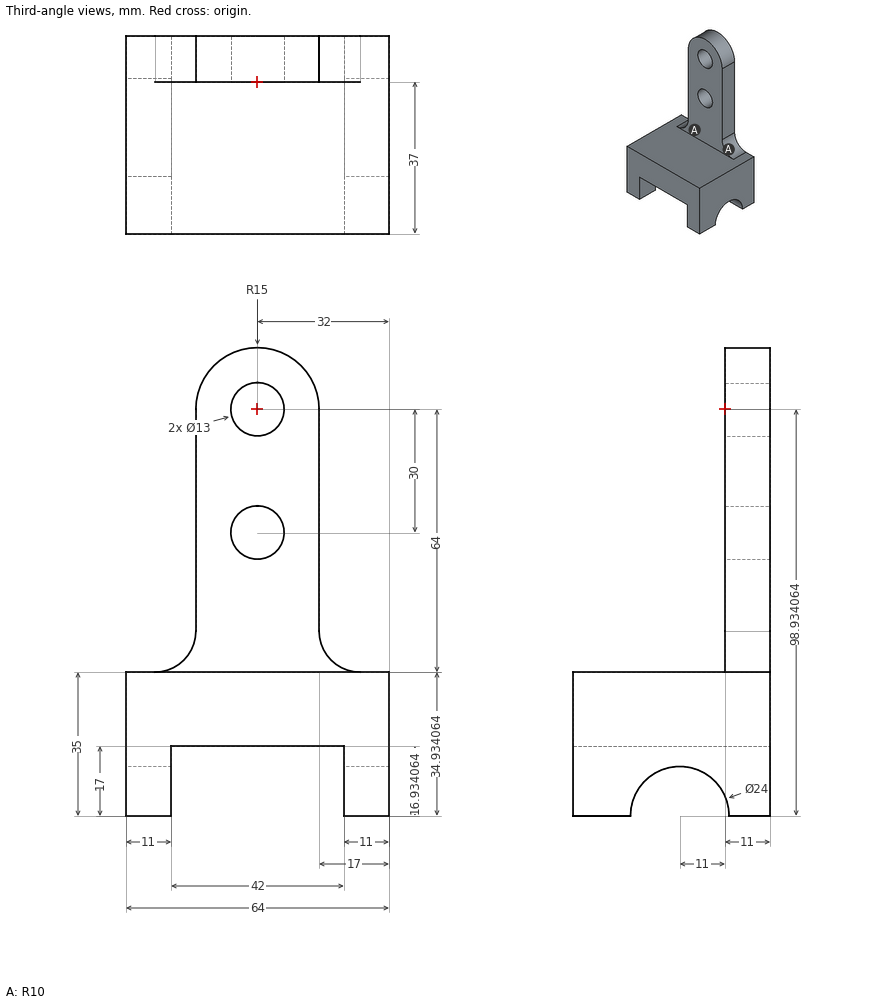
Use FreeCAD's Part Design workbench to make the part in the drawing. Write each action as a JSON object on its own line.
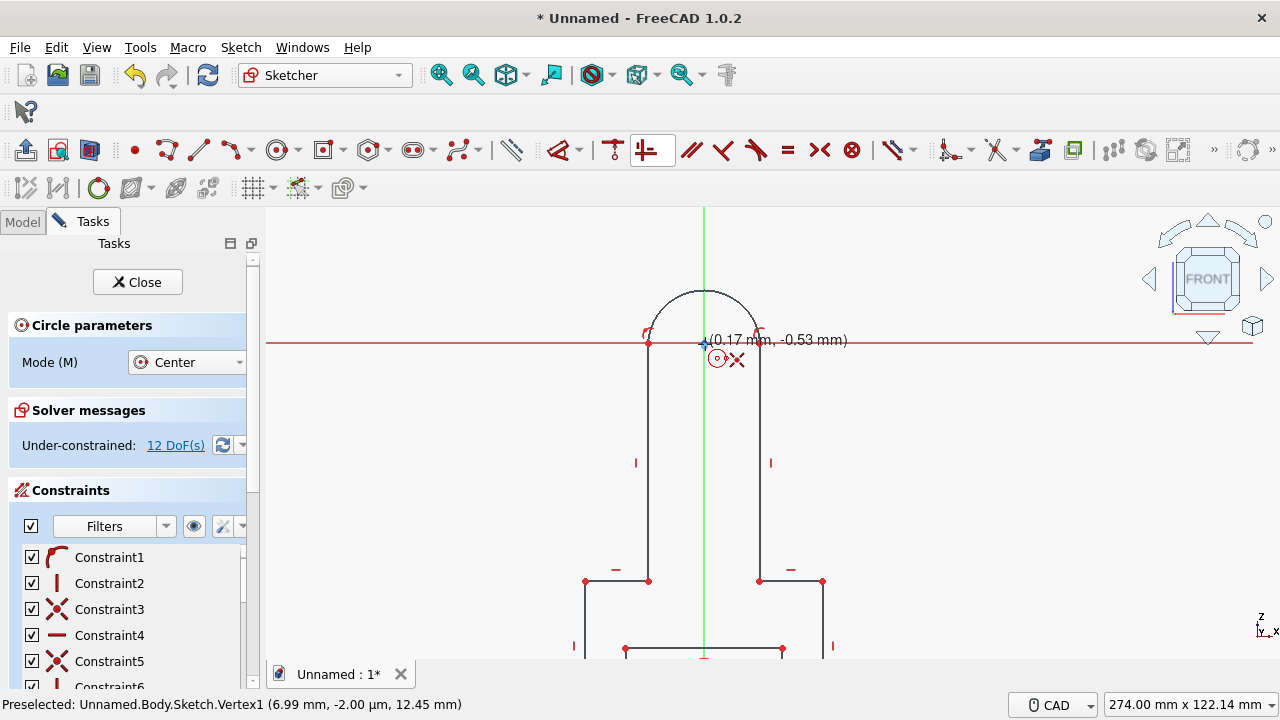
{"action": "left_click", "coordinate": [704, 343]}
{"action": "left_click", "coordinate": [721, 326]}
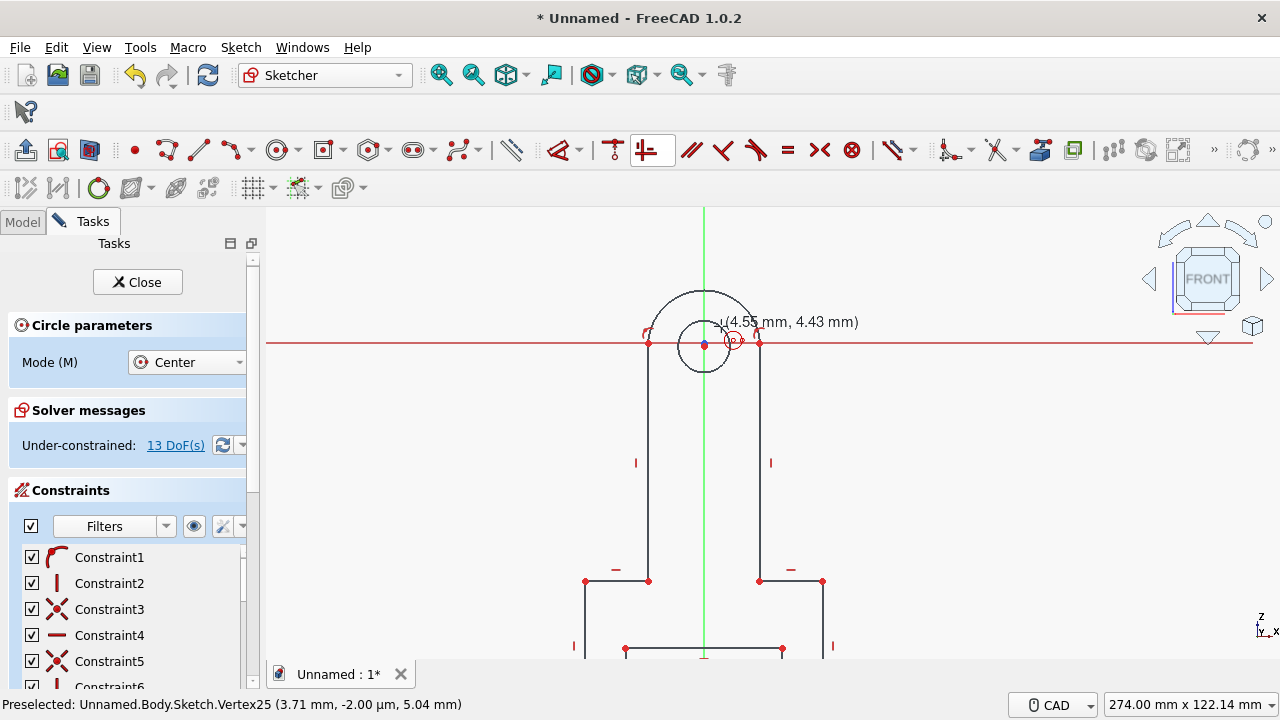
{"action": "left_click", "coordinate": [704, 454]}
{"action": "left_click", "coordinate": [721, 437]}
{"action": "key", "text": "Escape"}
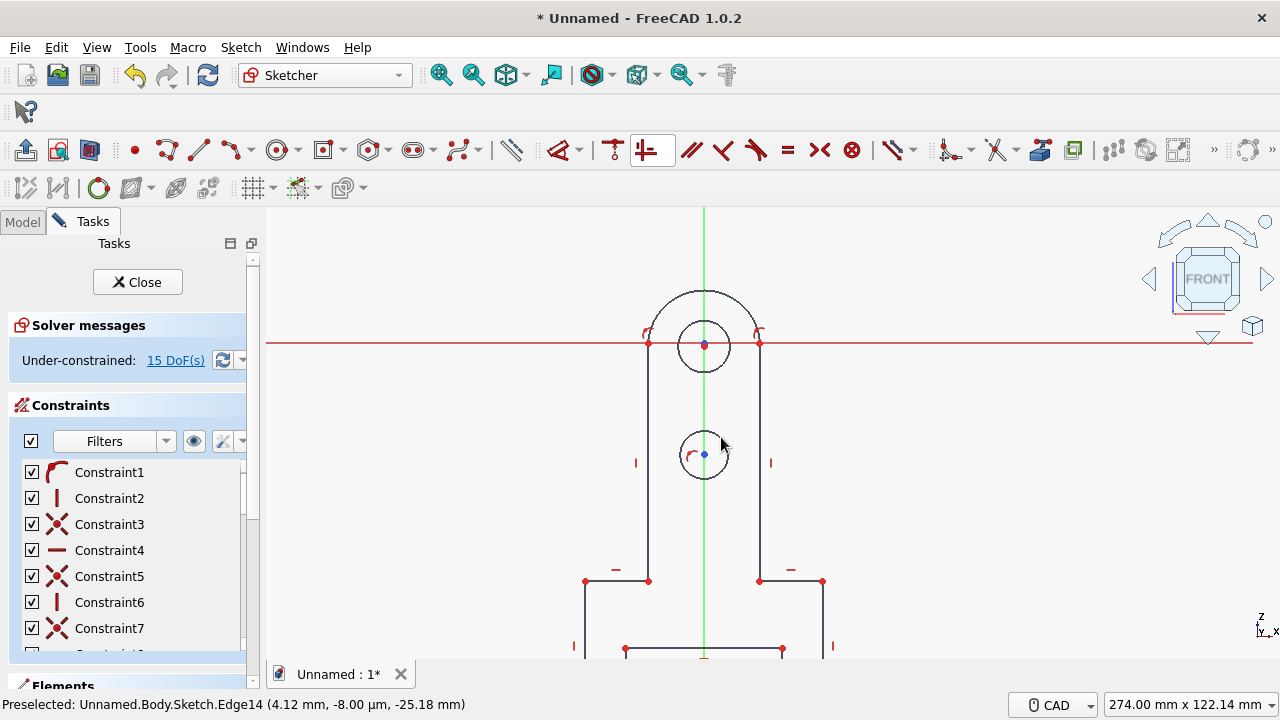
{"action": "left_click", "coordinate": [760, 415]}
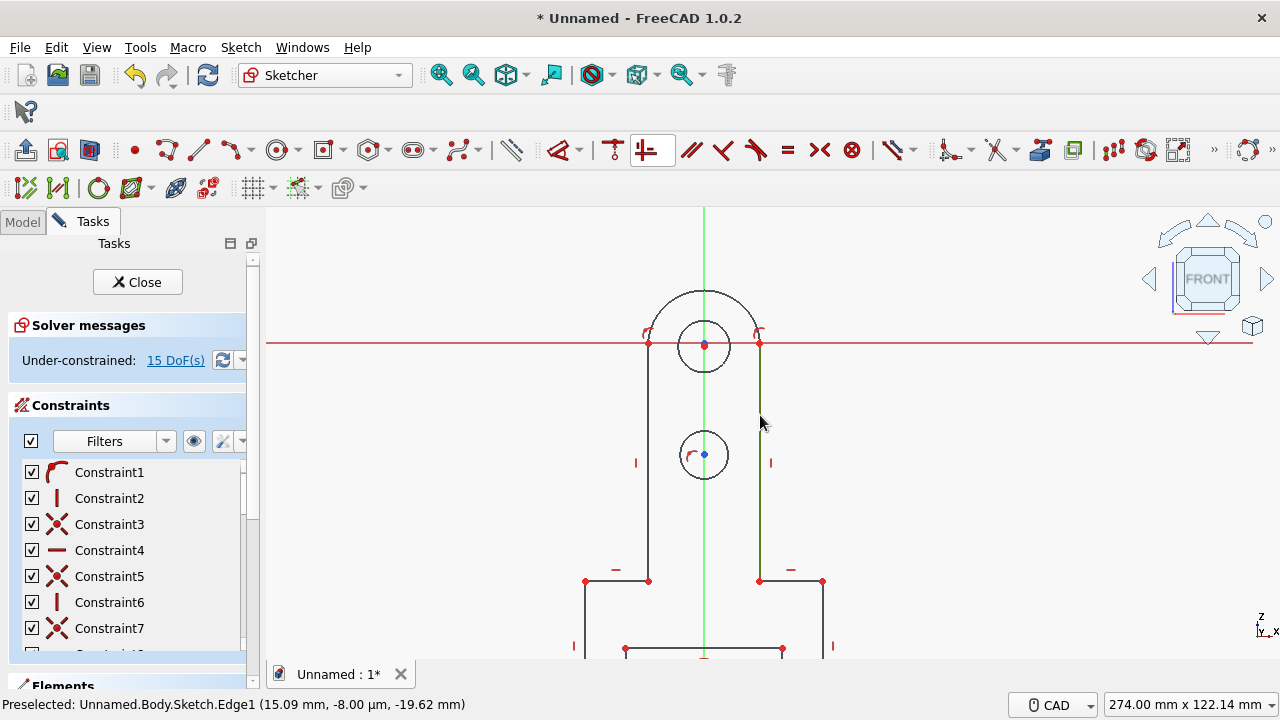
{"action": "left_click", "coordinate": [736, 300]}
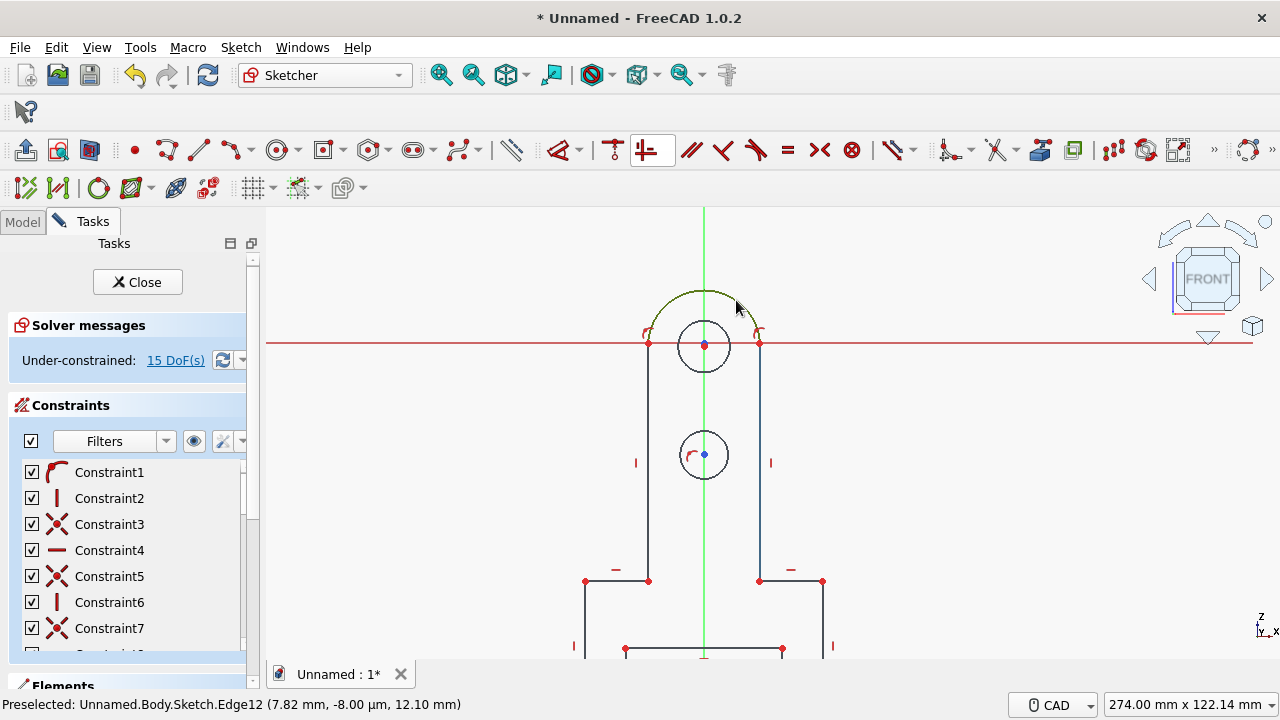
{"action": "left_click", "coordinate": [756, 150]}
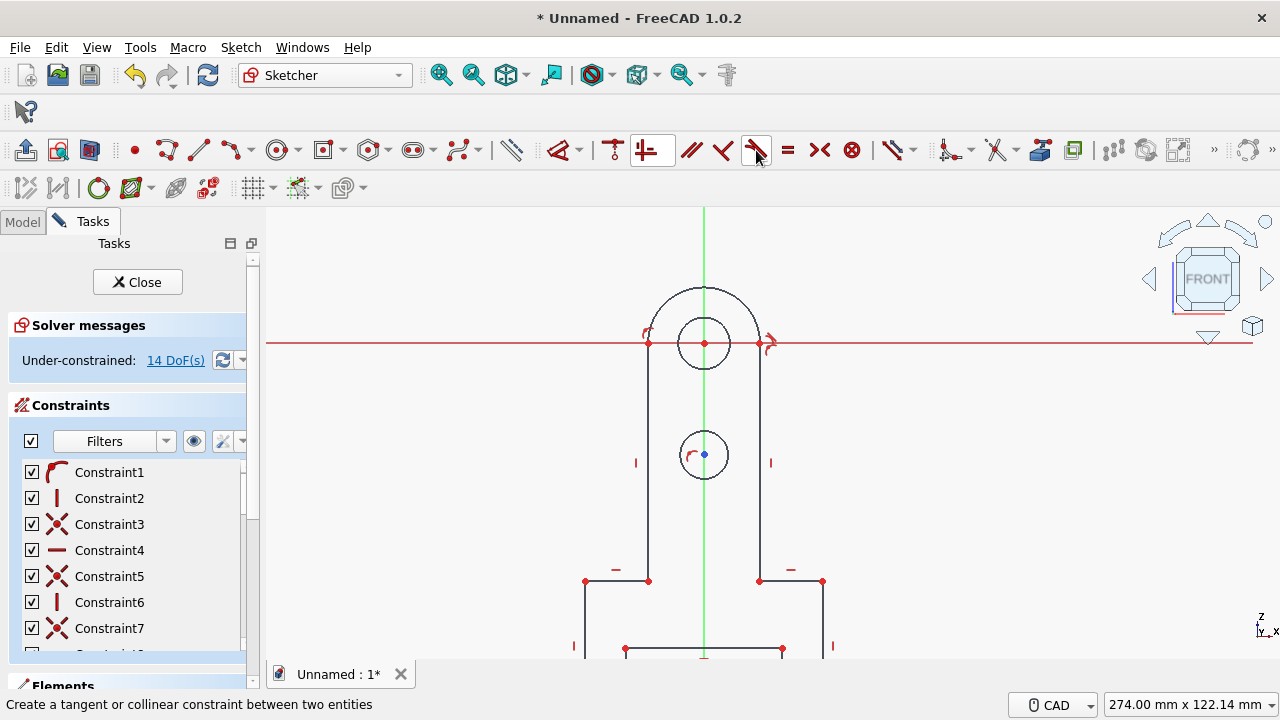
{"action": "left_click", "coordinate": [722, 325]}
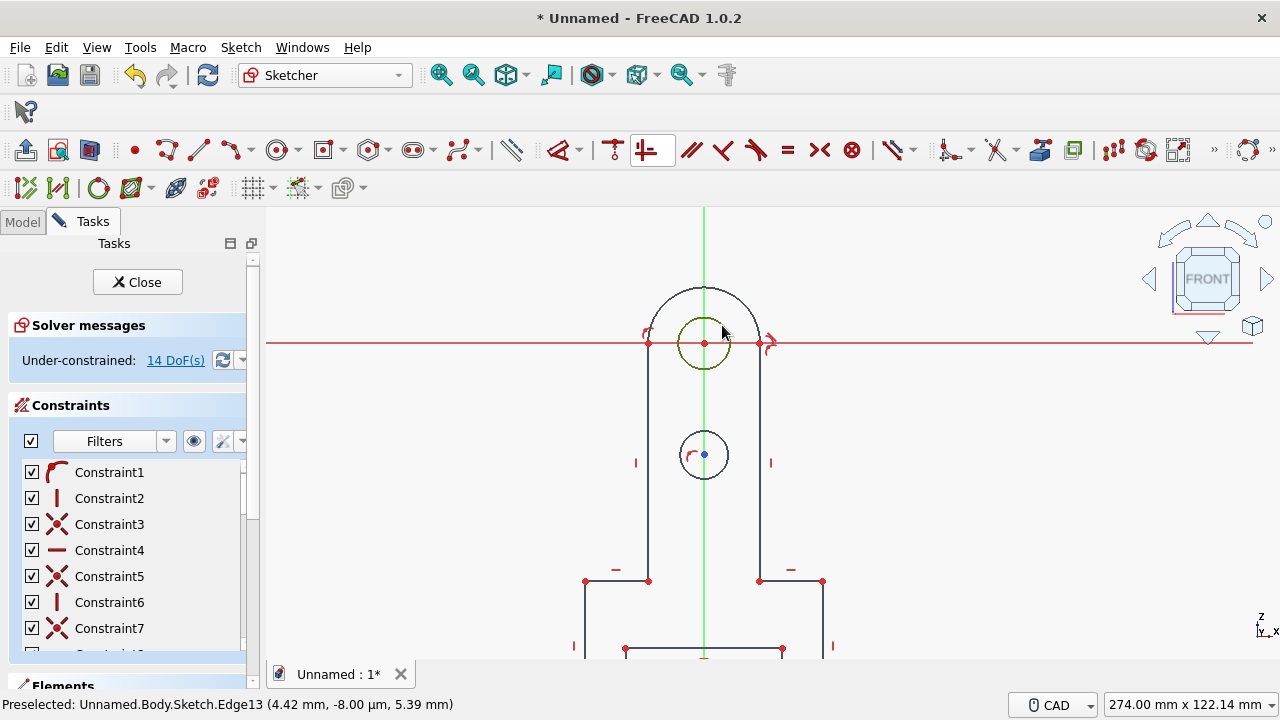
{"action": "left_click", "coordinate": [721, 438]}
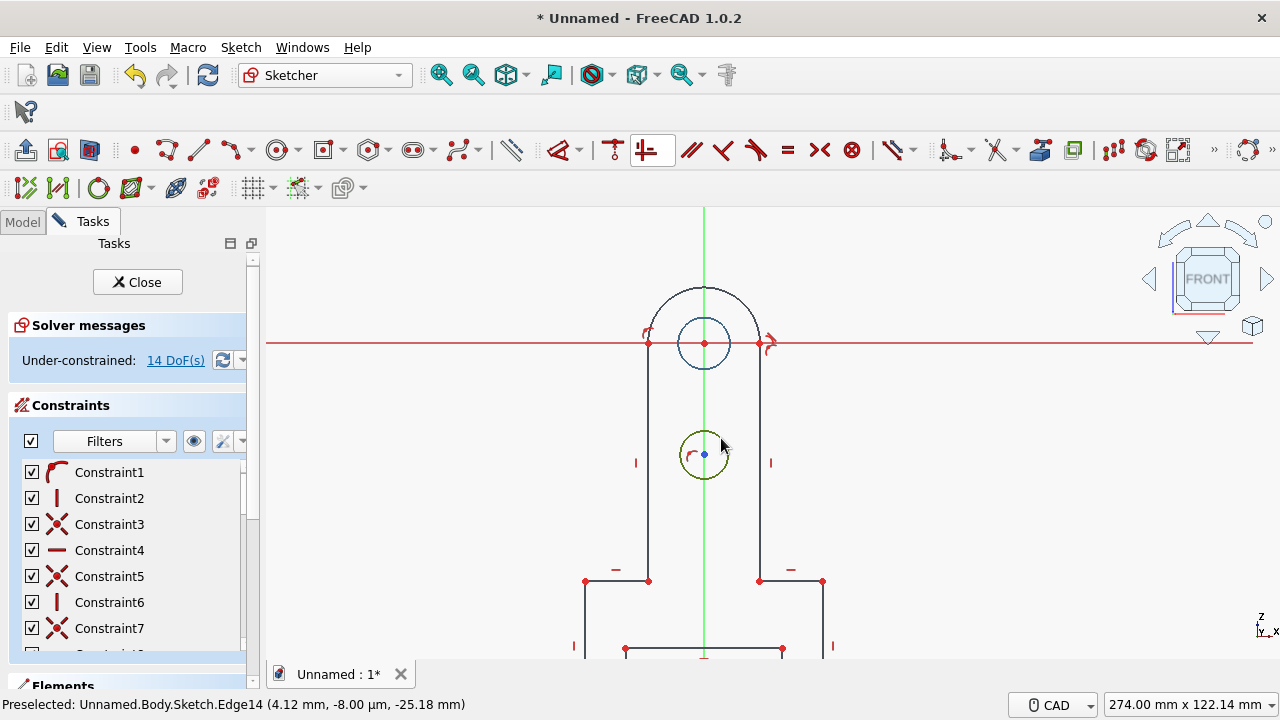
{"action": "left_click", "coordinate": [788, 150]}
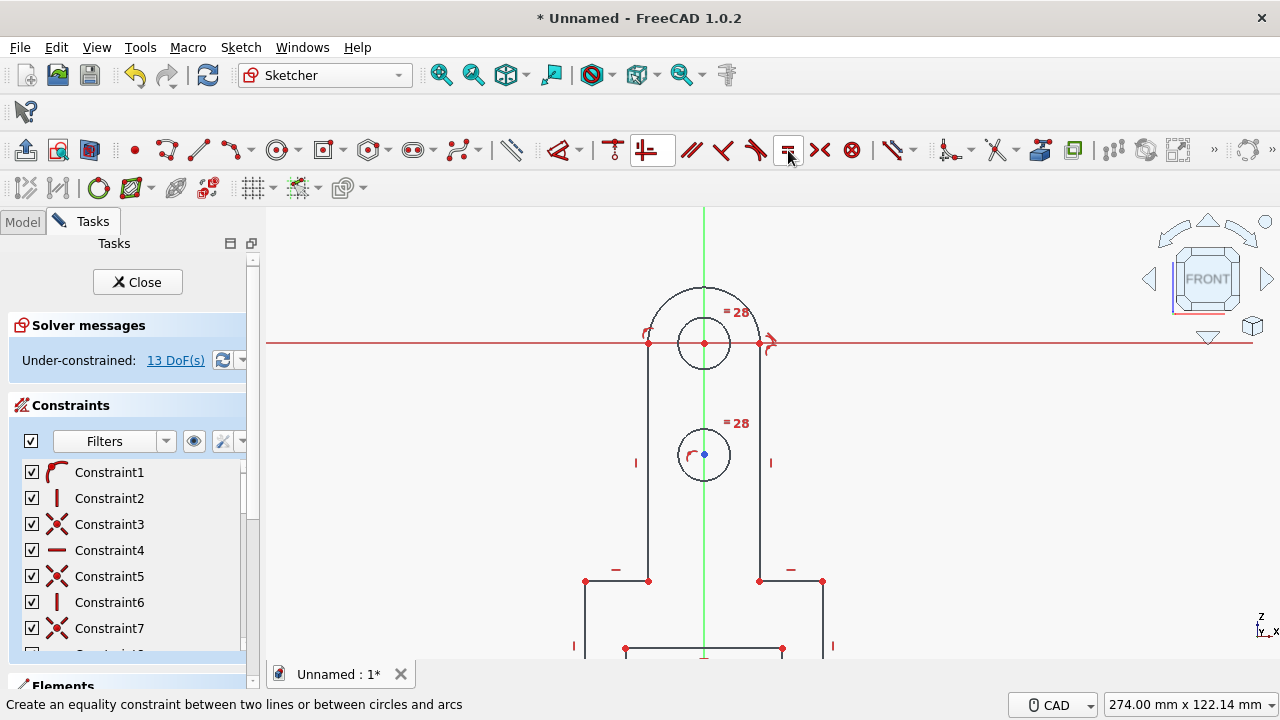
{"action": "left_click", "coordinate": [704, 343]}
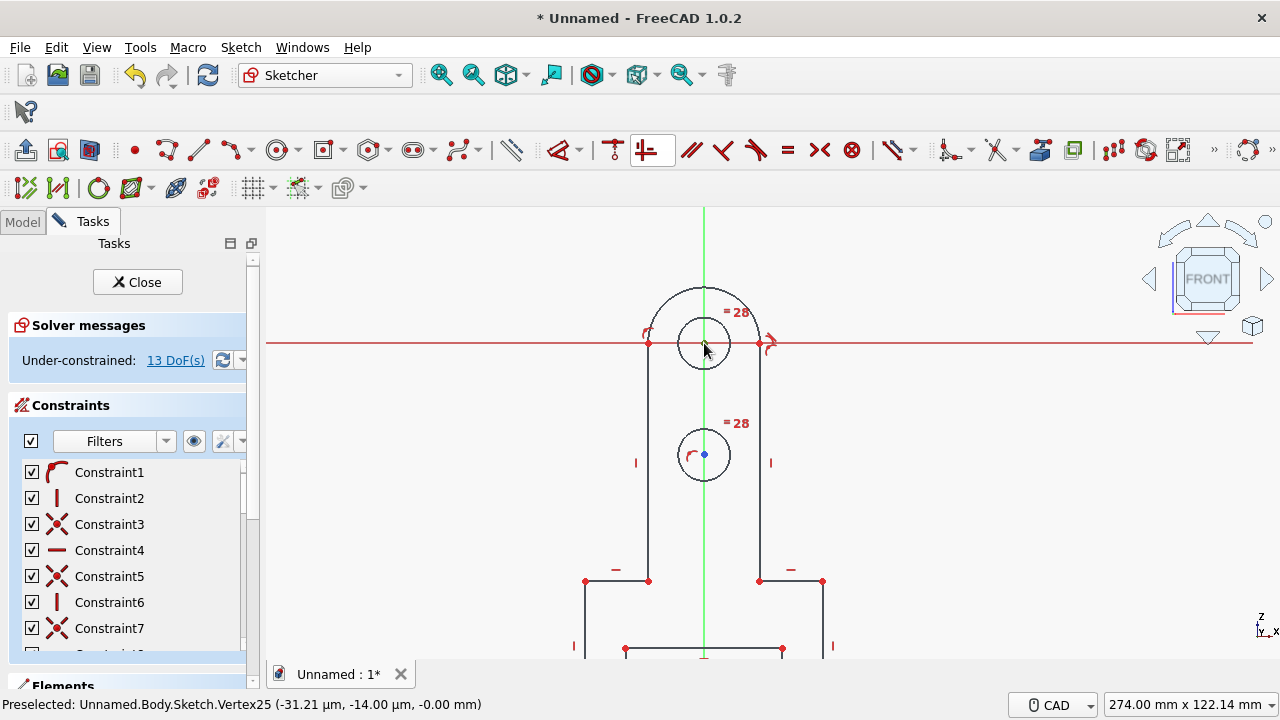
{"action": "left_click", "coordinate": [704, 603]}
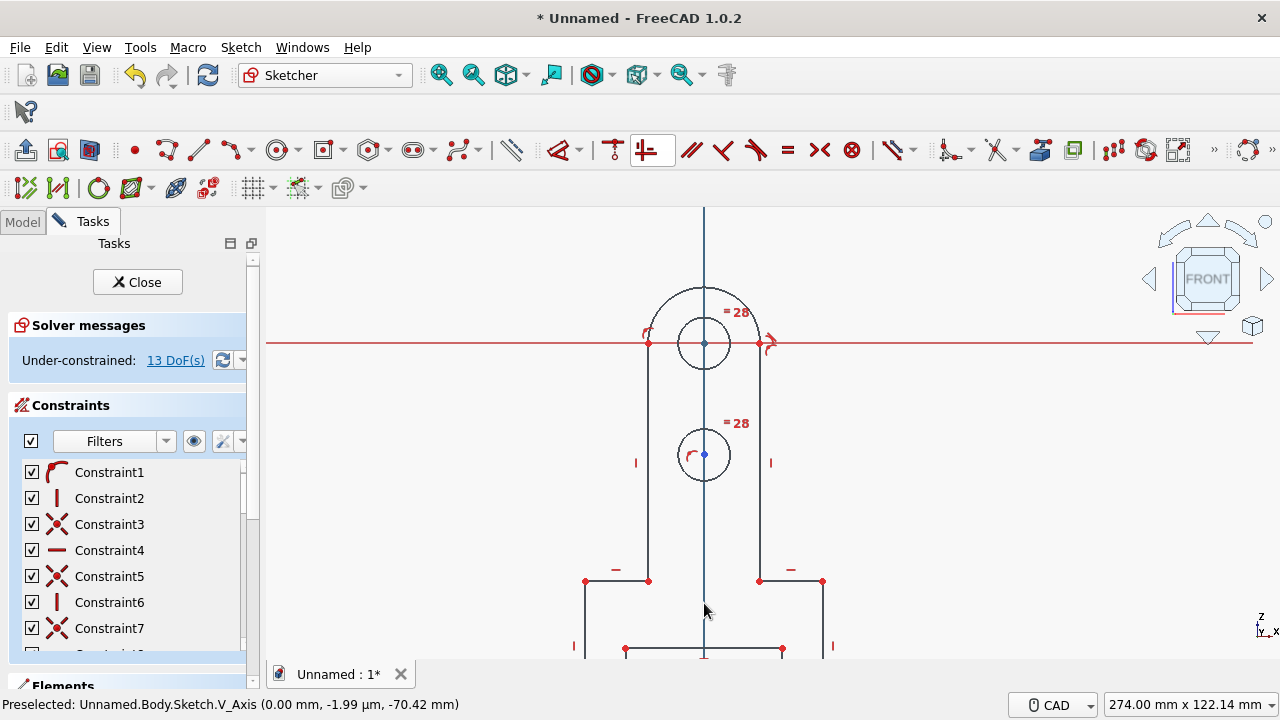
{"action": "left_click", "coordinate": [614, 150]}